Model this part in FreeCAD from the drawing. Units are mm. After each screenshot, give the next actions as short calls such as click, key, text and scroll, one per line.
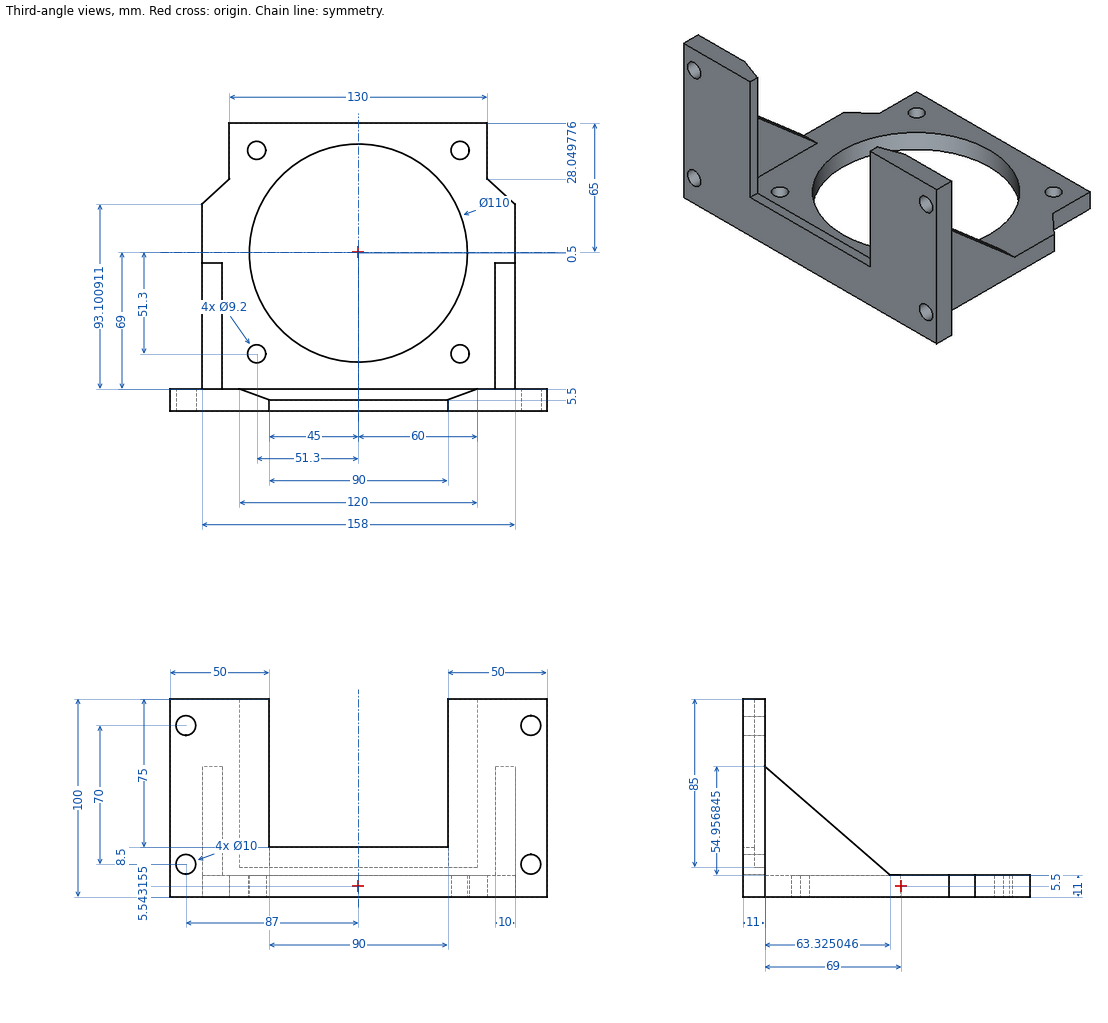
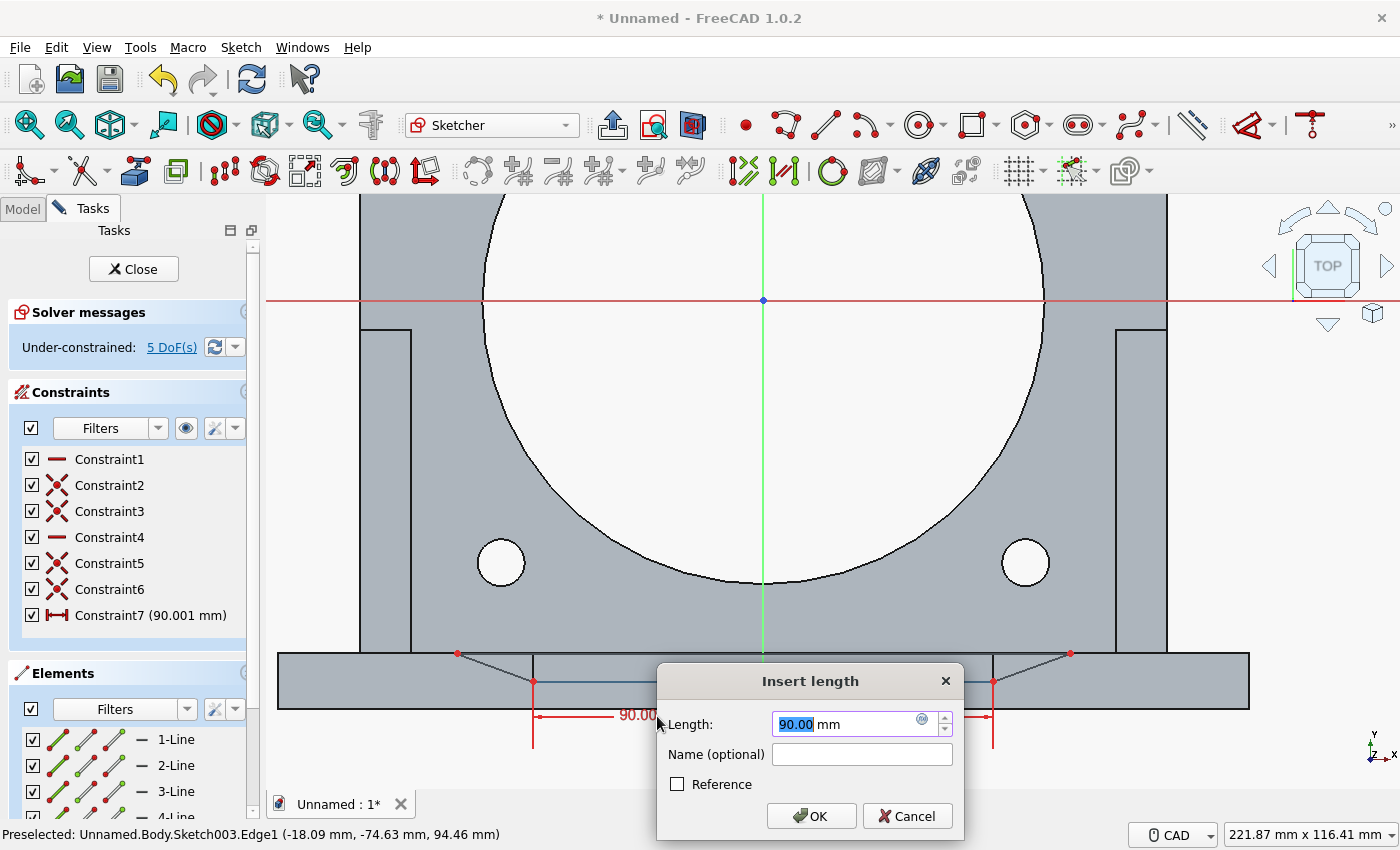
text(90)
key(Return)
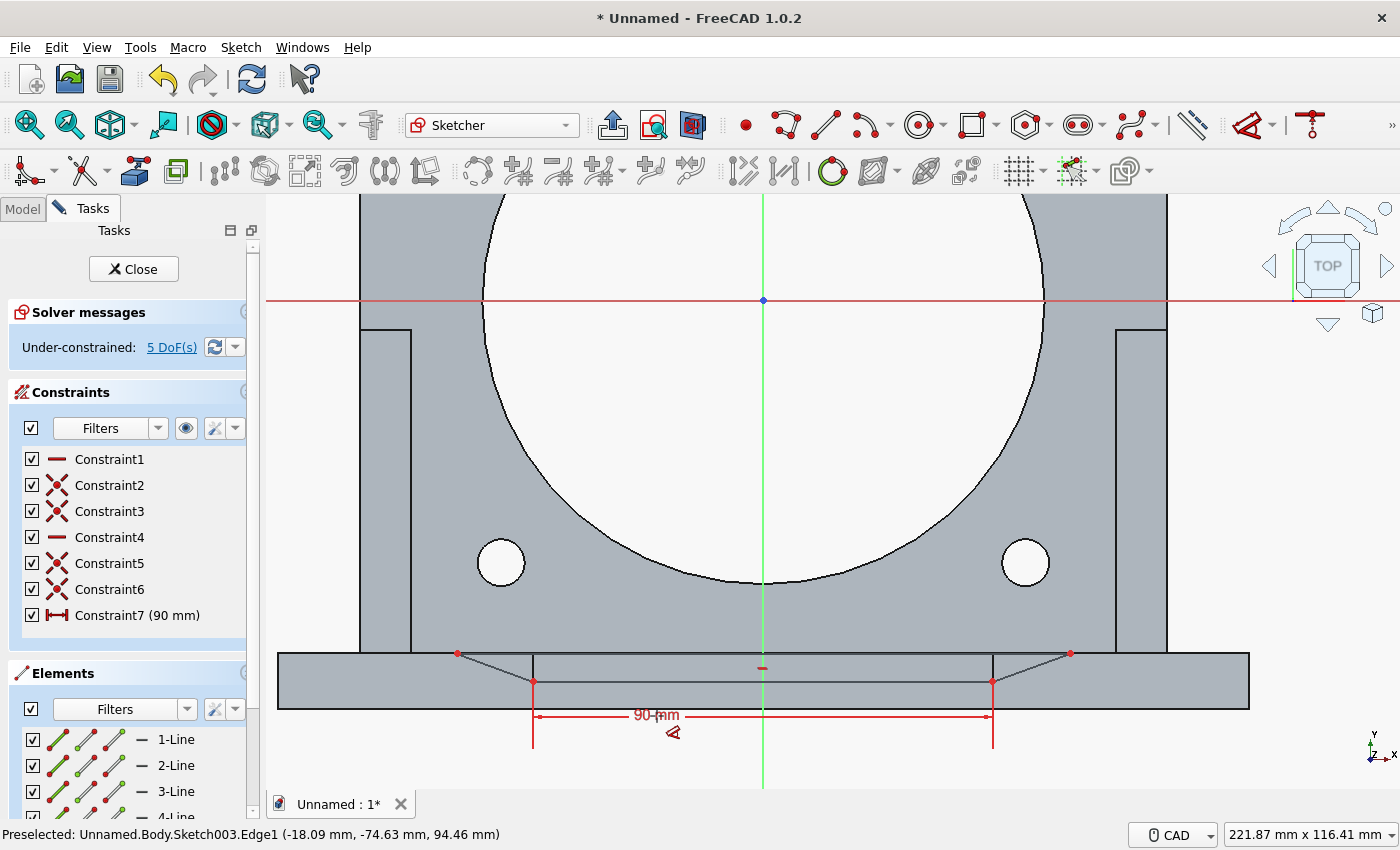
click(886, 654)
click(623, 620)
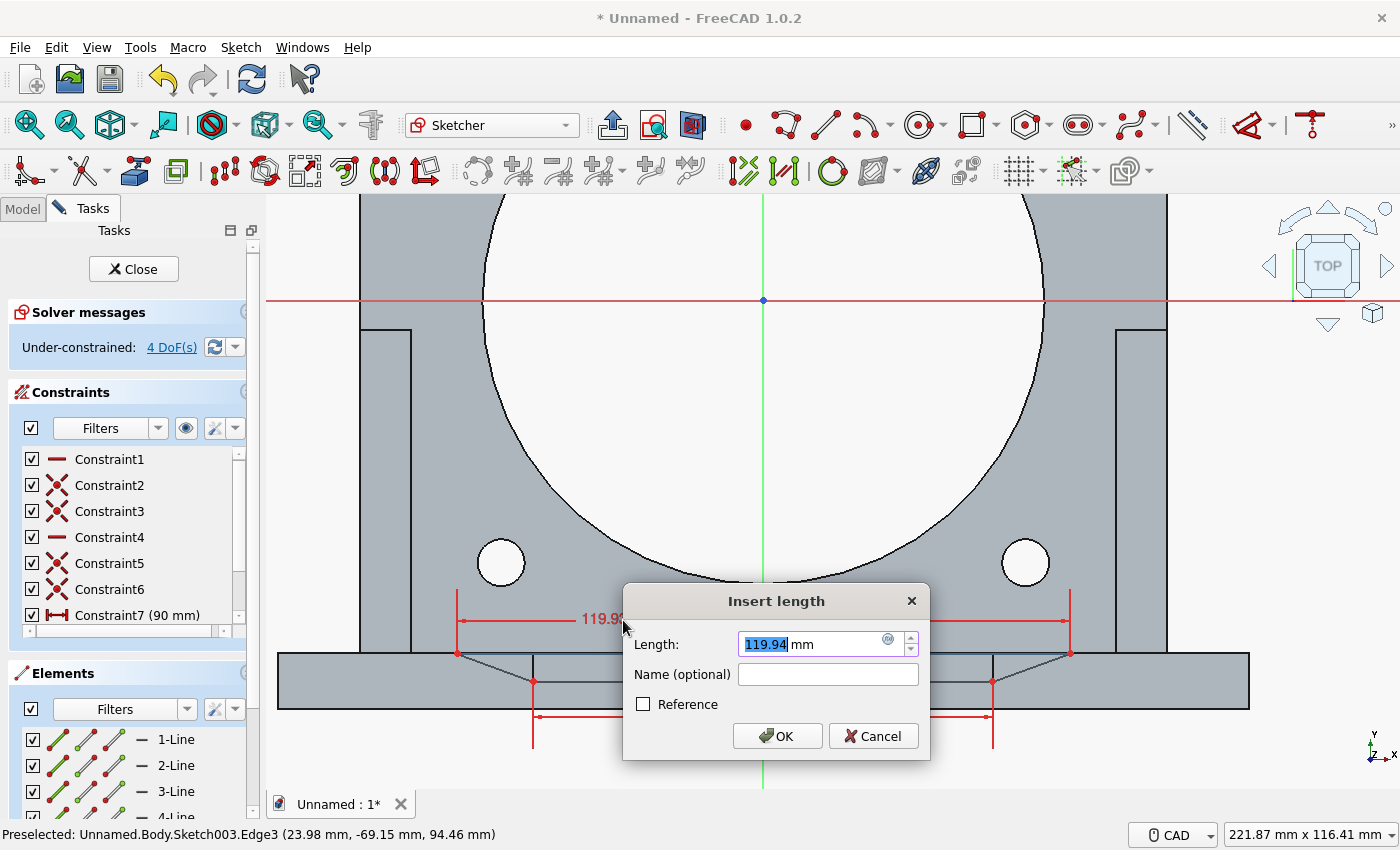
text(120)
key(Return)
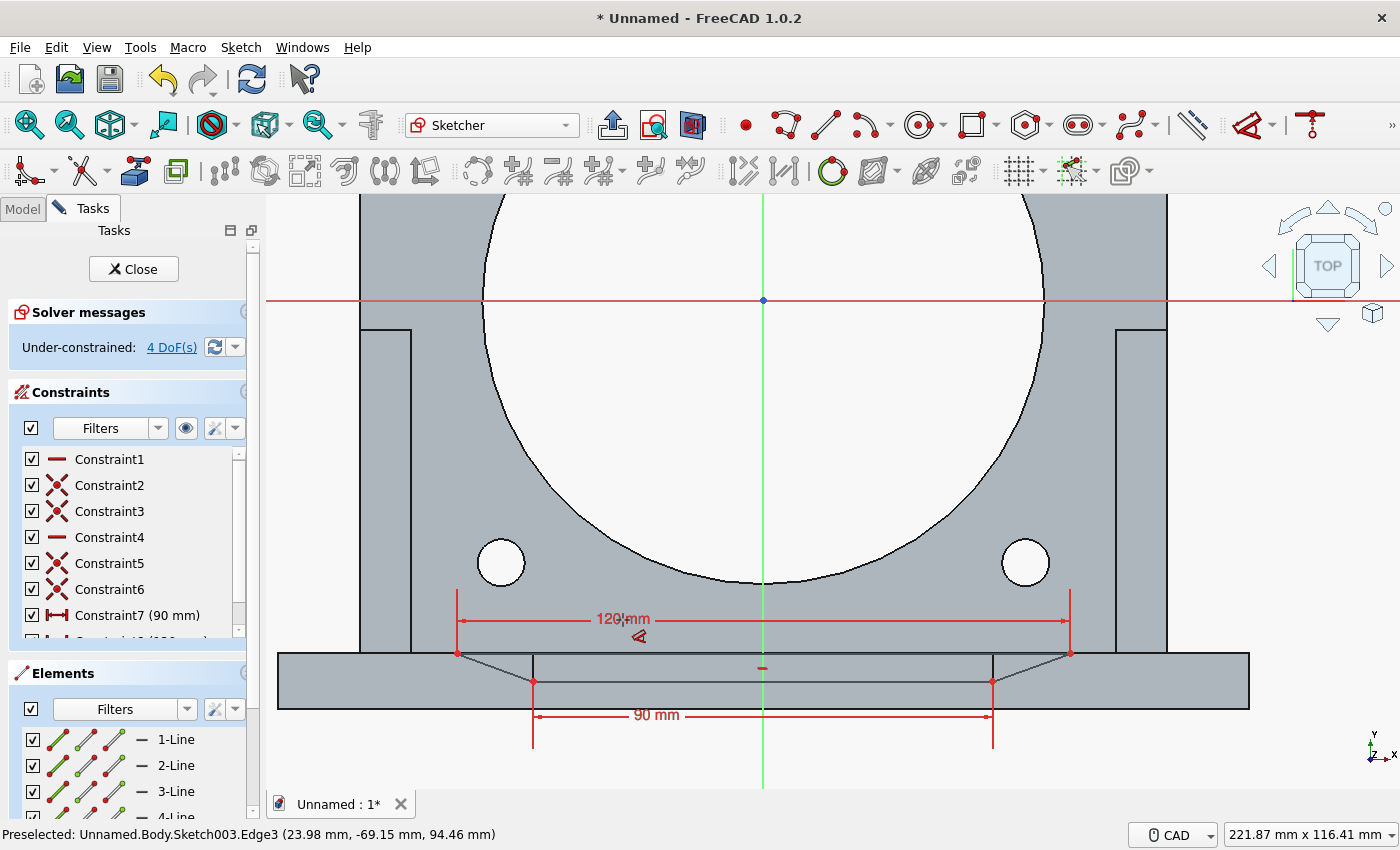
click(533, 682)
click(568, 716)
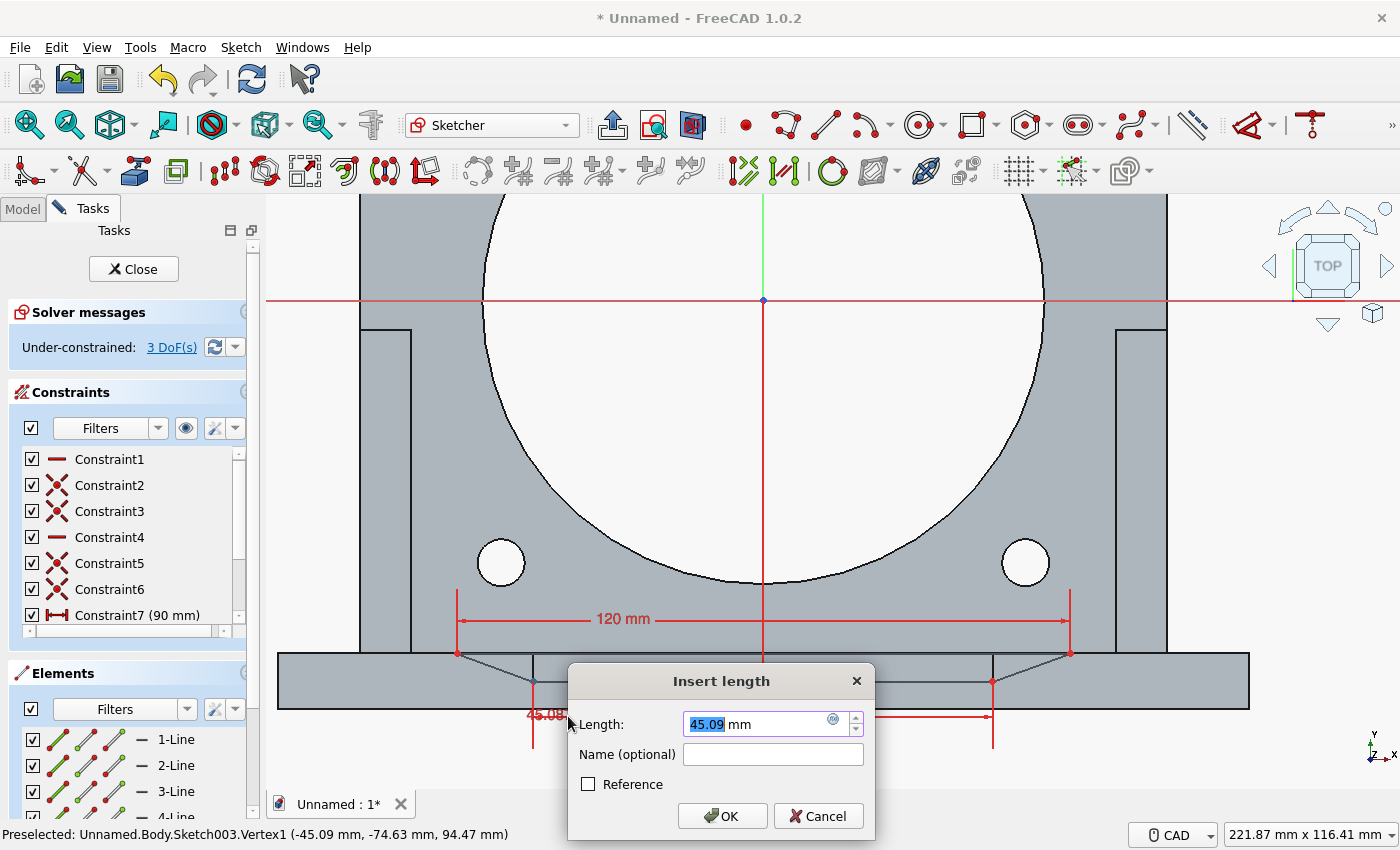
text(45)
key(Return)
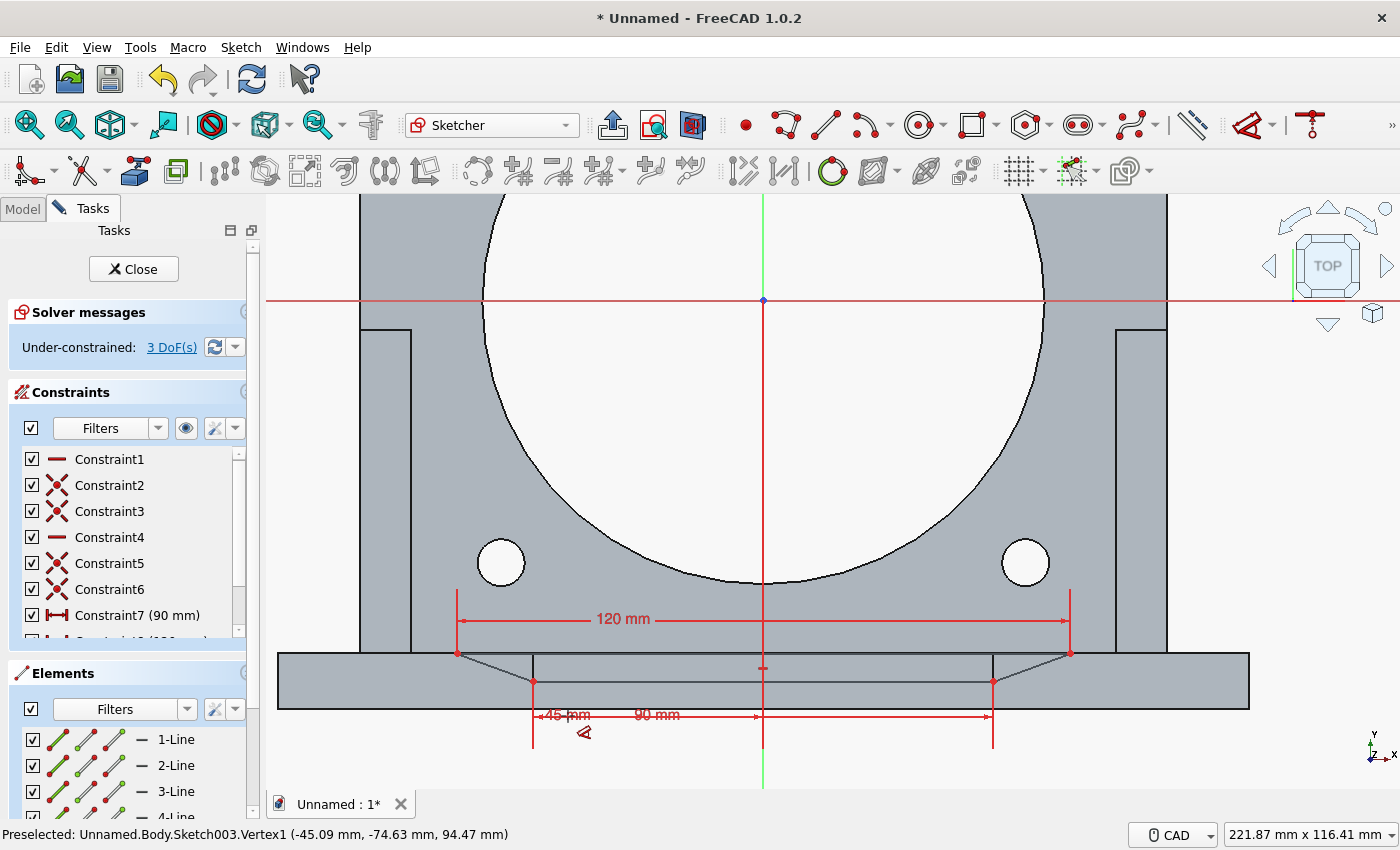
click(1070, 654)
click(917, 267)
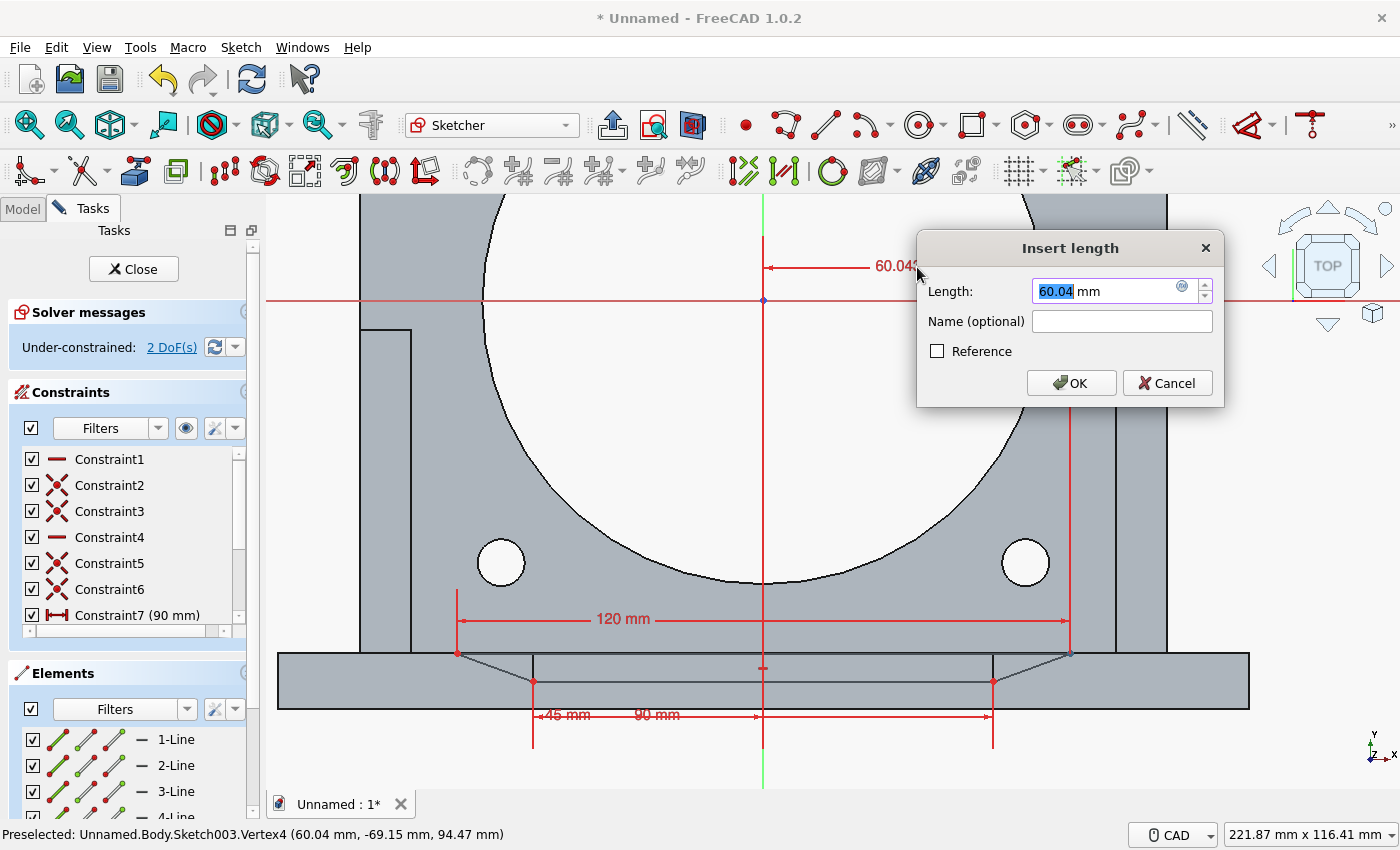
text(60)
key(Return)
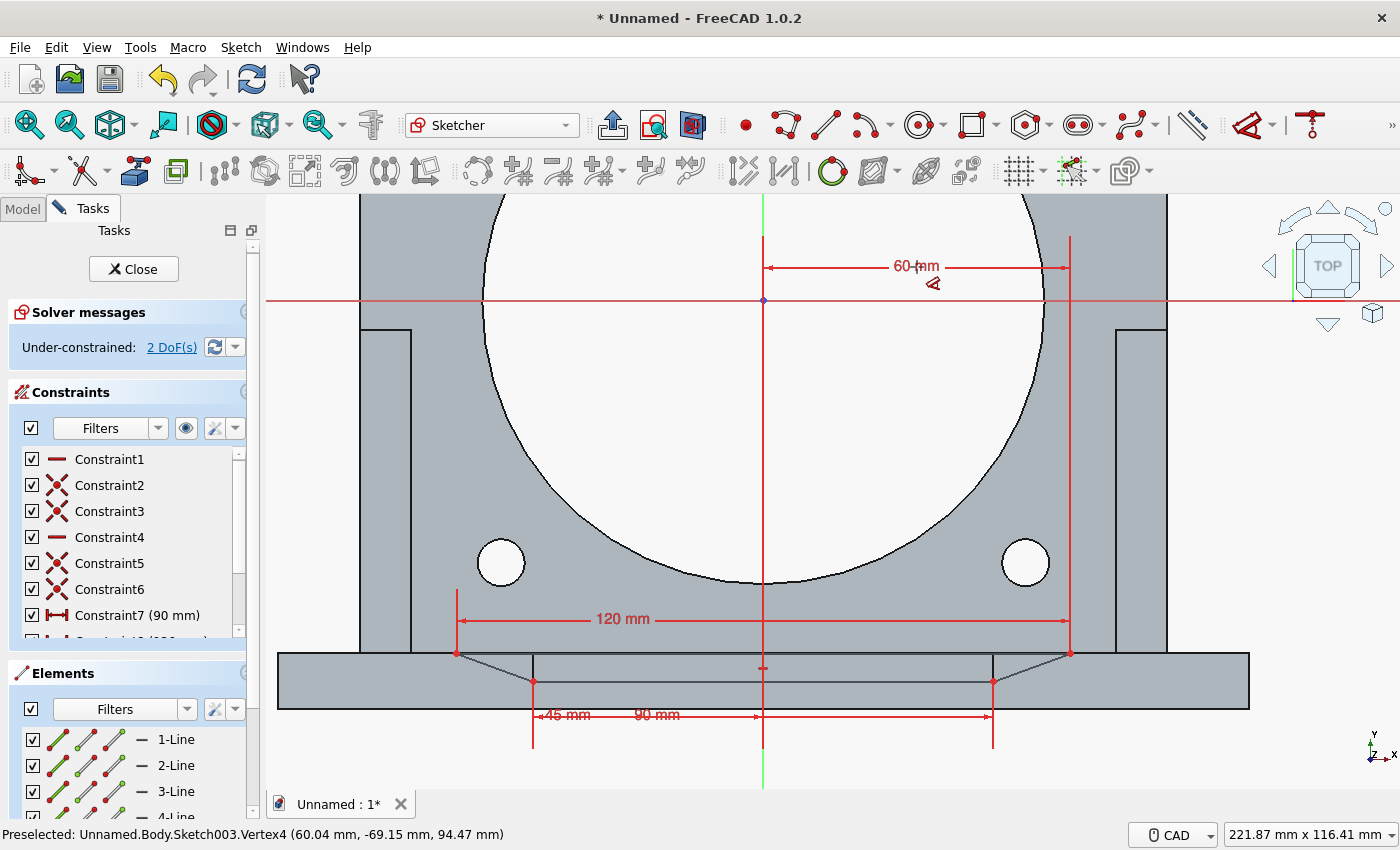
click(1070, 654)
click(1104, 477)